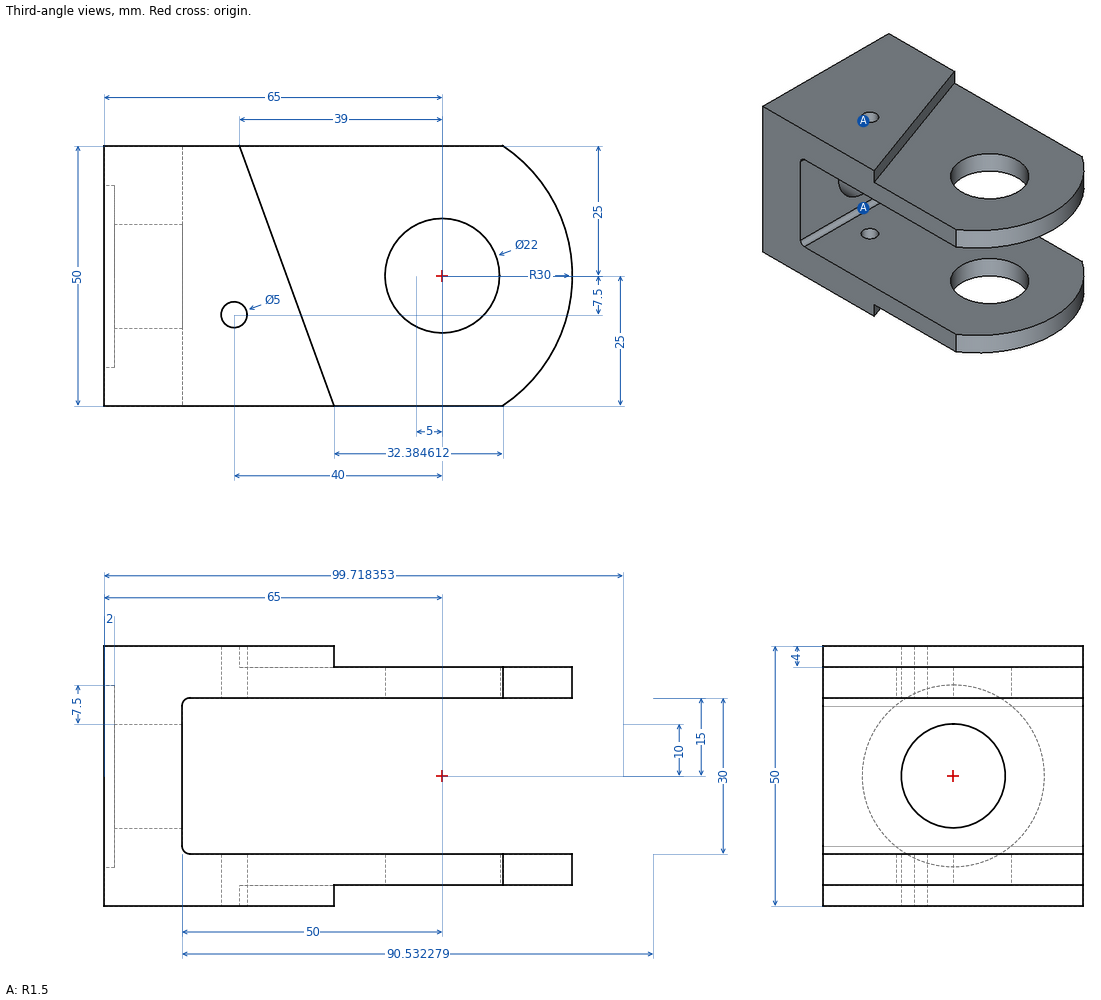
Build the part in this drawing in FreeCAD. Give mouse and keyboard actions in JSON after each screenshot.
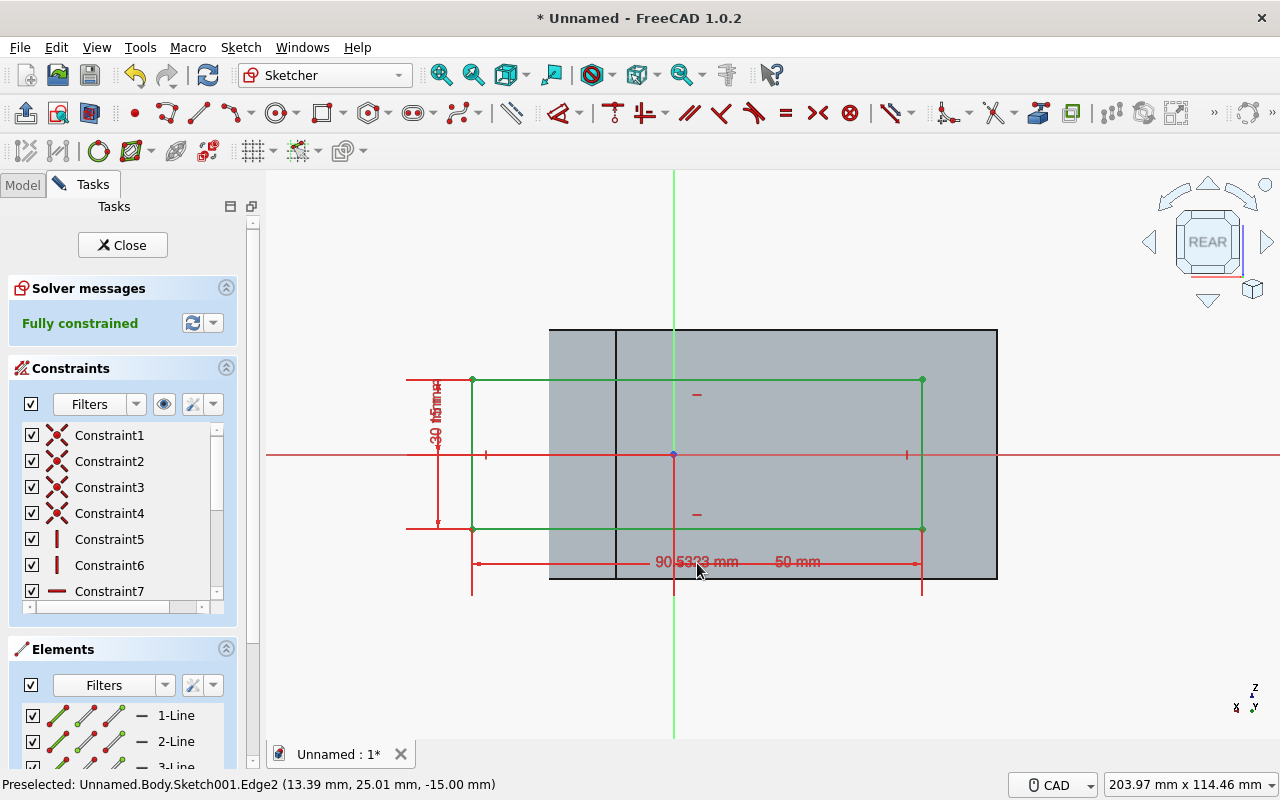
{"action": "left_click", "coordinate": [123, 245]}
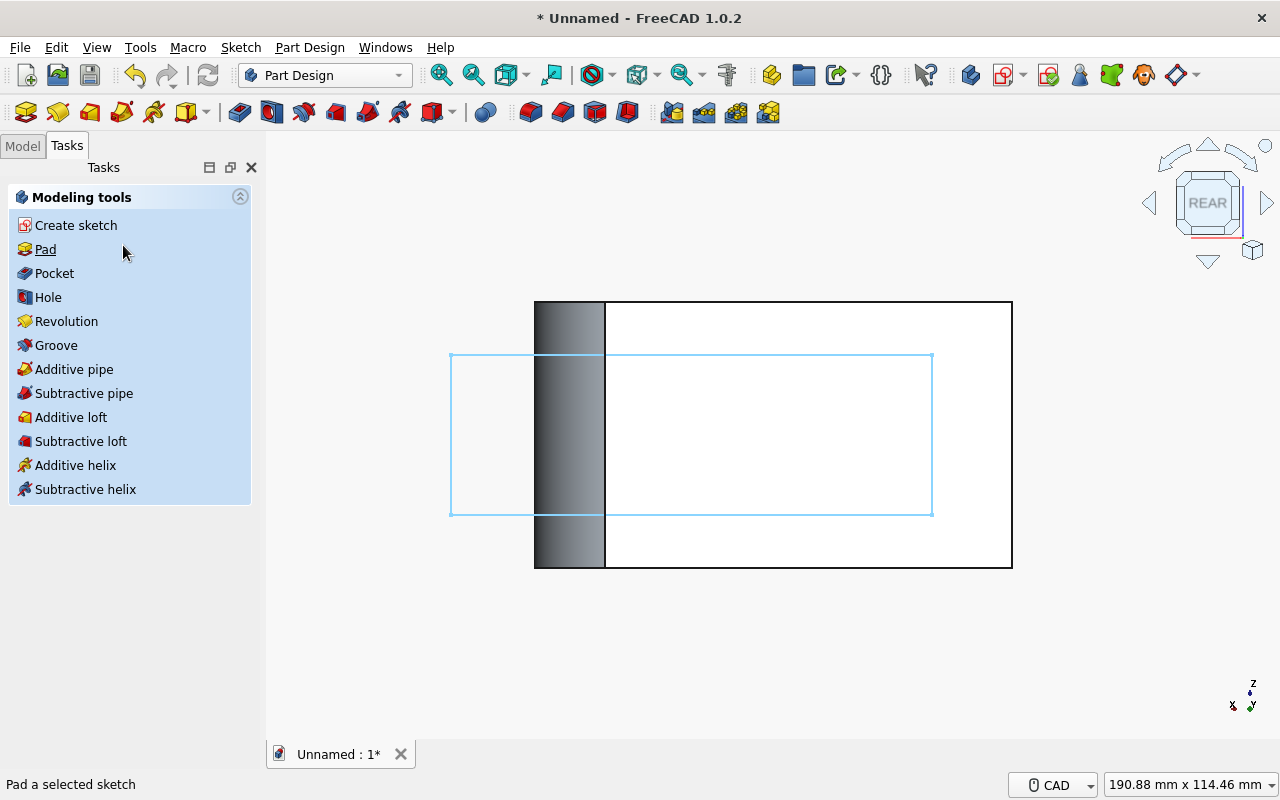
{"action": "left_click", "coordinate": [240, 112]}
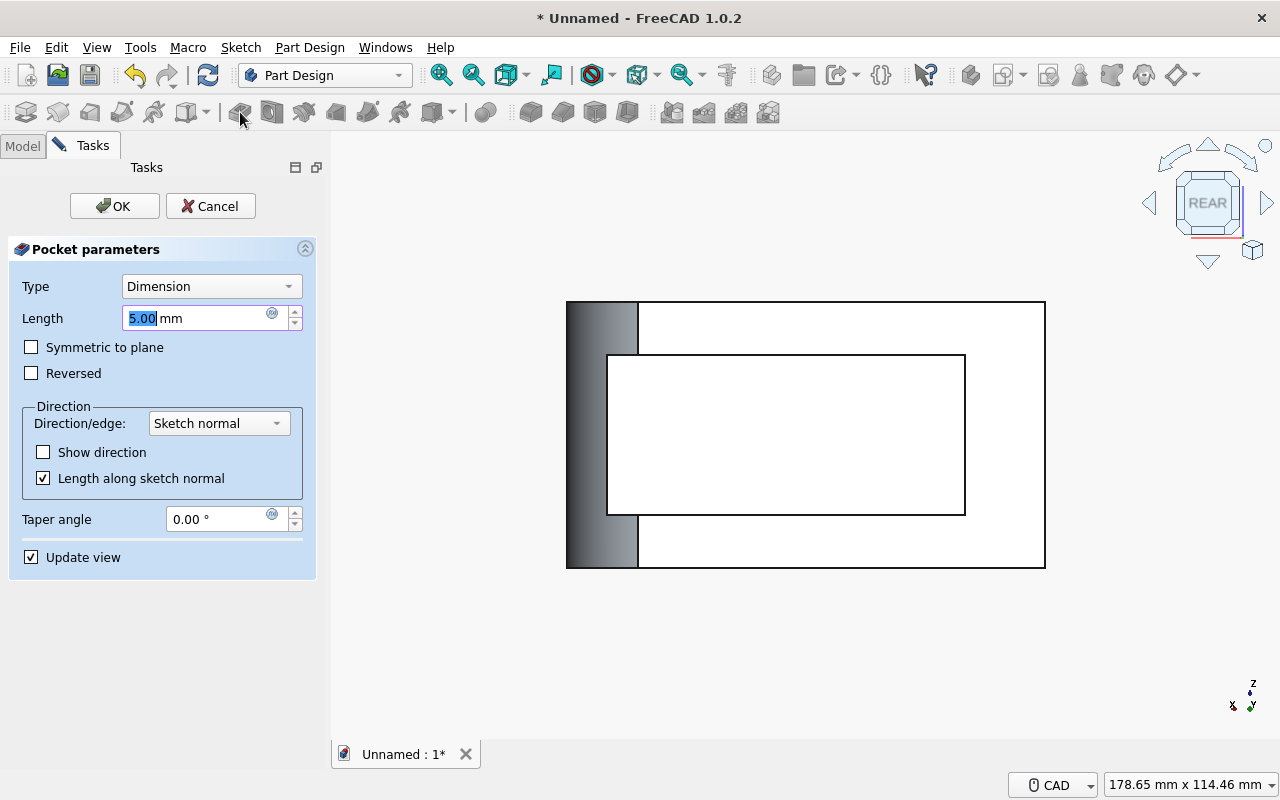
{"action": "left_click", "coordinate": [212, 286]}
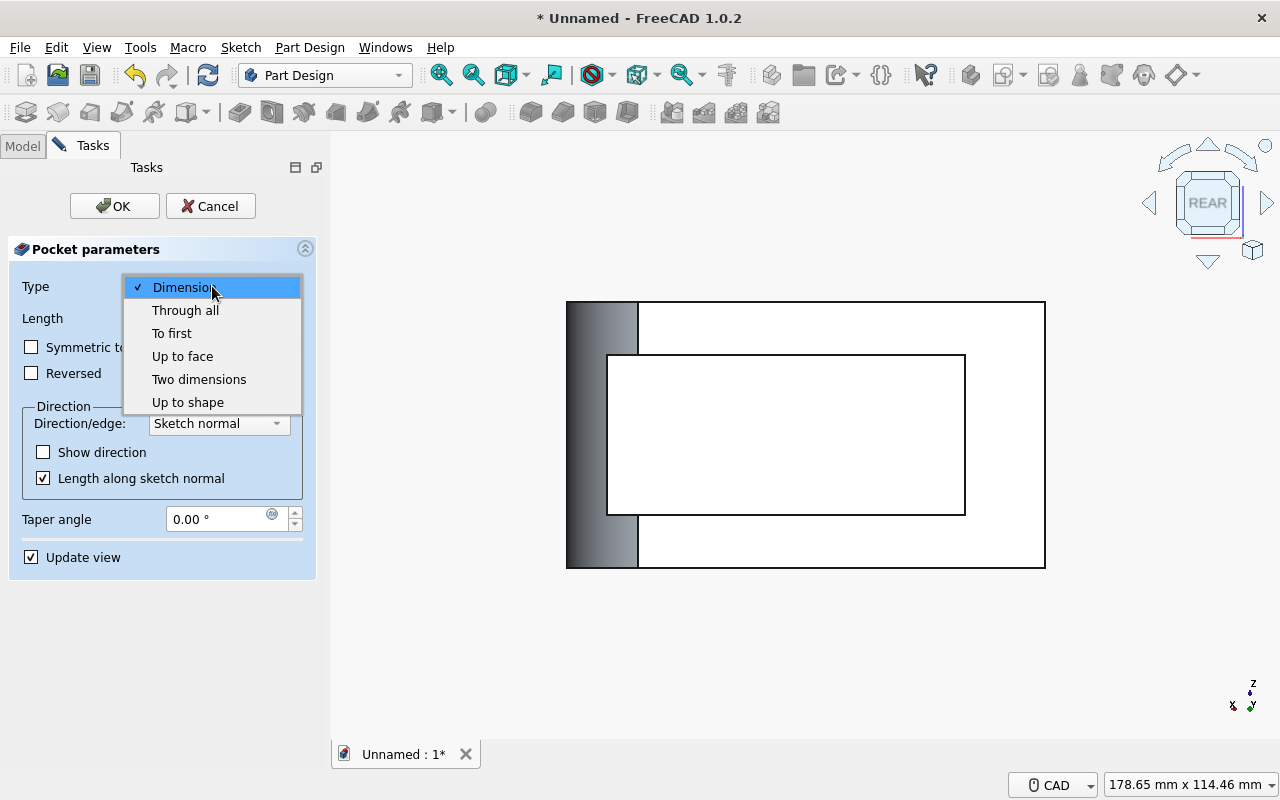
{"action": "left_click", "coordinate": [212, 310]}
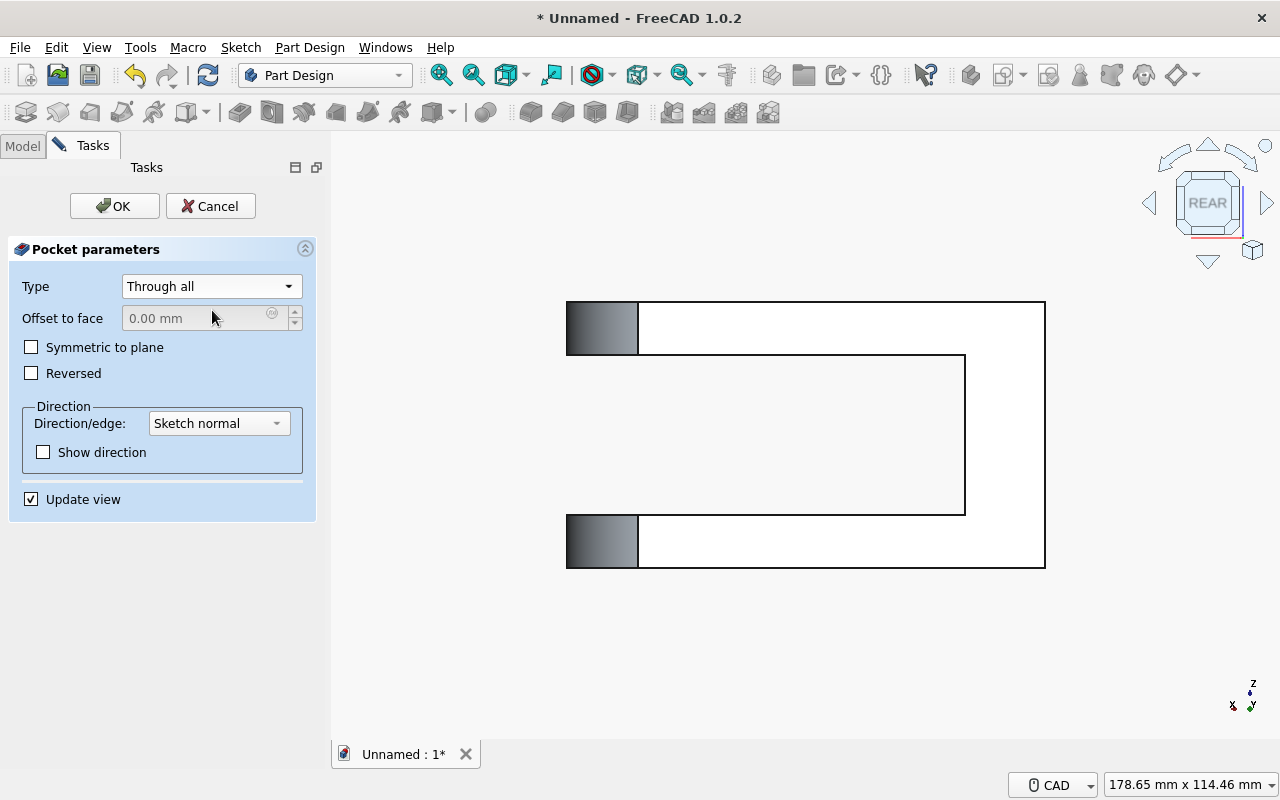
{"action": "left_click", "coordinate": [115, 206]}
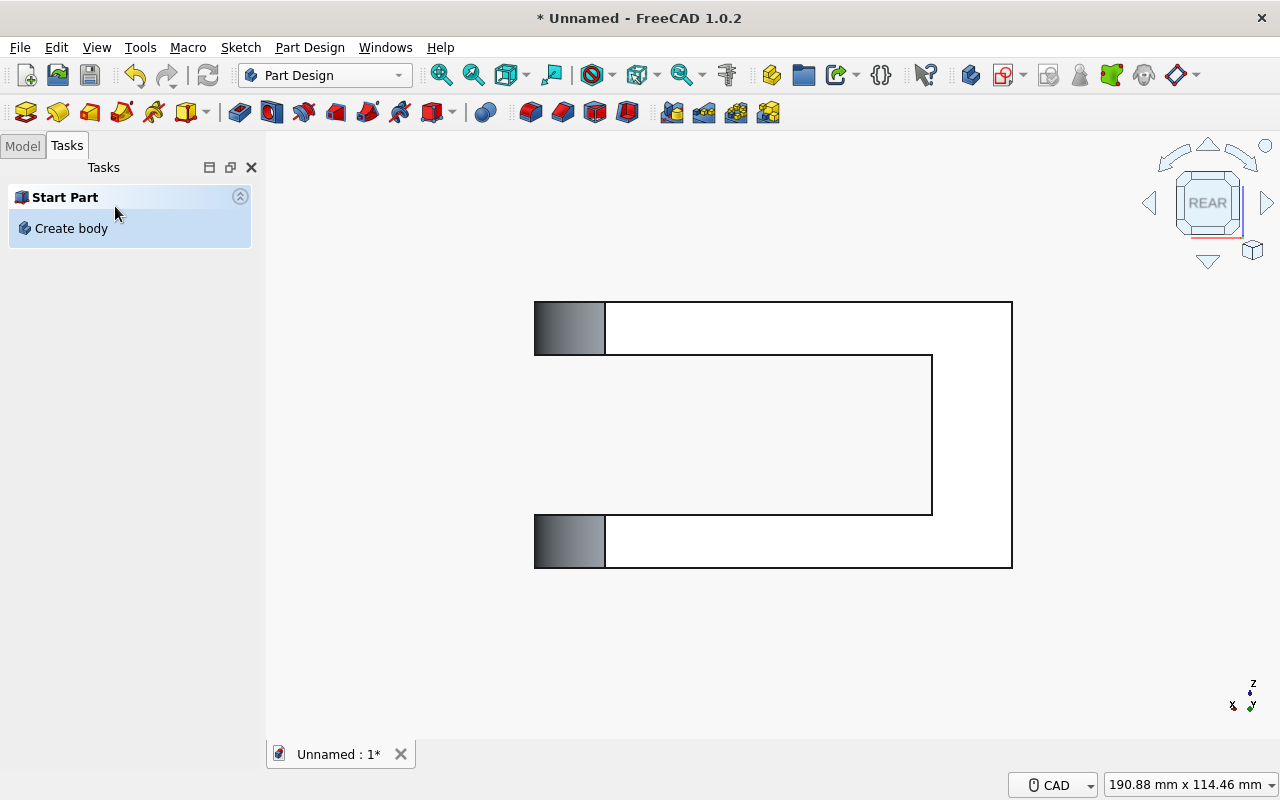
{"action": "key", "text": "0"}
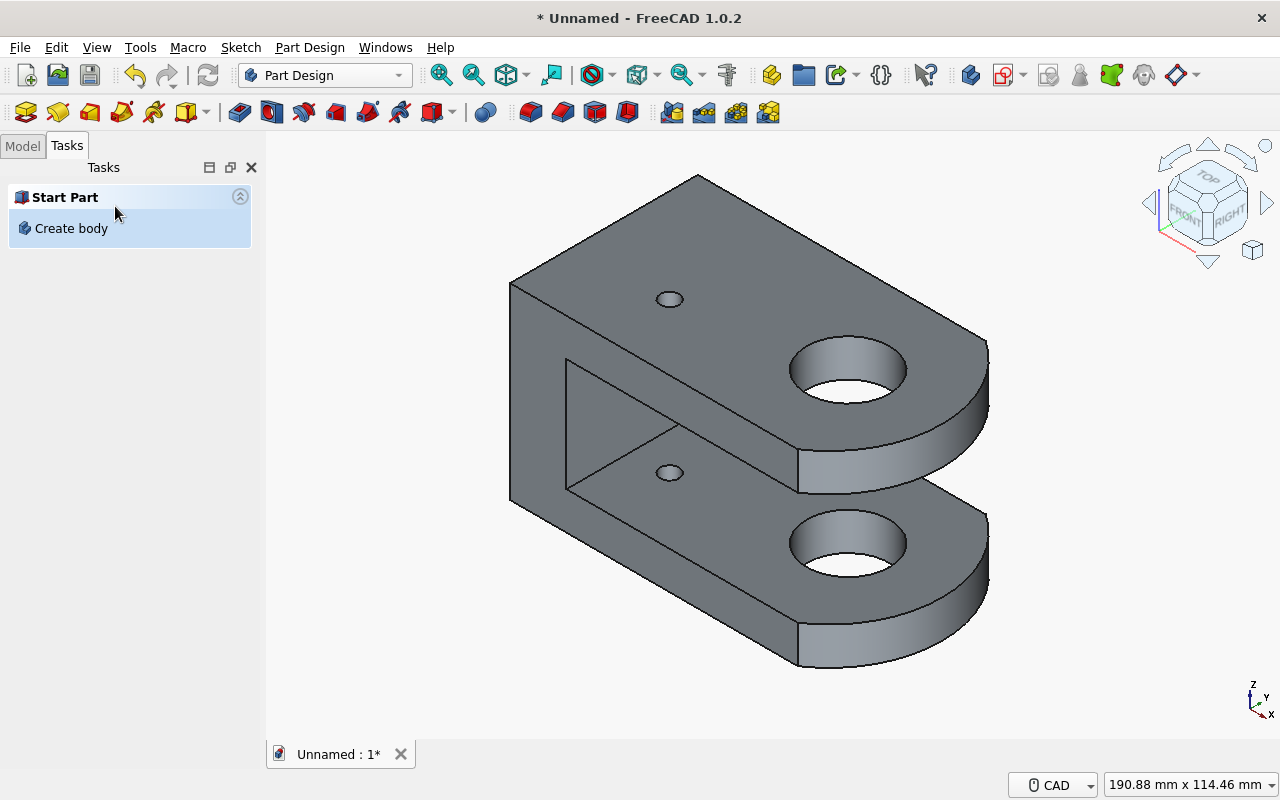
{"action": "left_click", "coordinate": [752, 282]}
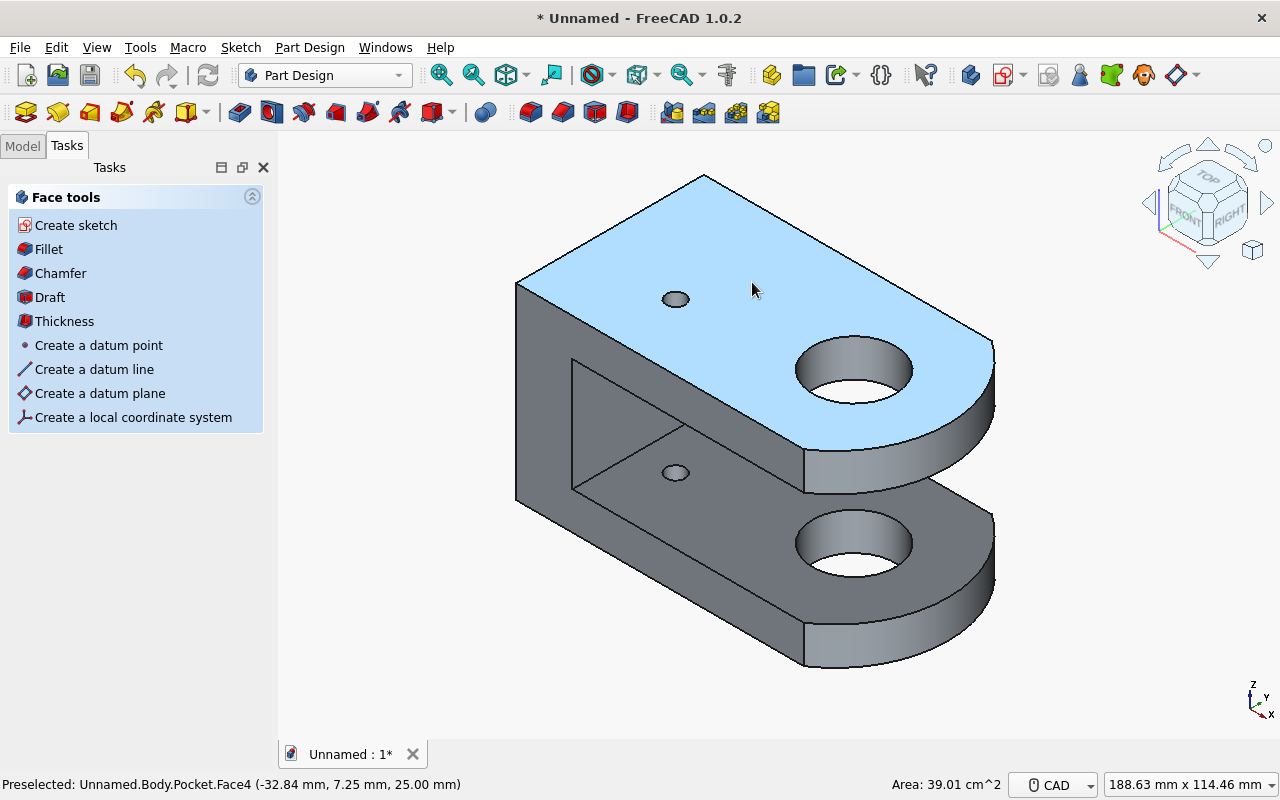
{"action": "left_click", "coordinate": [1004, 76]}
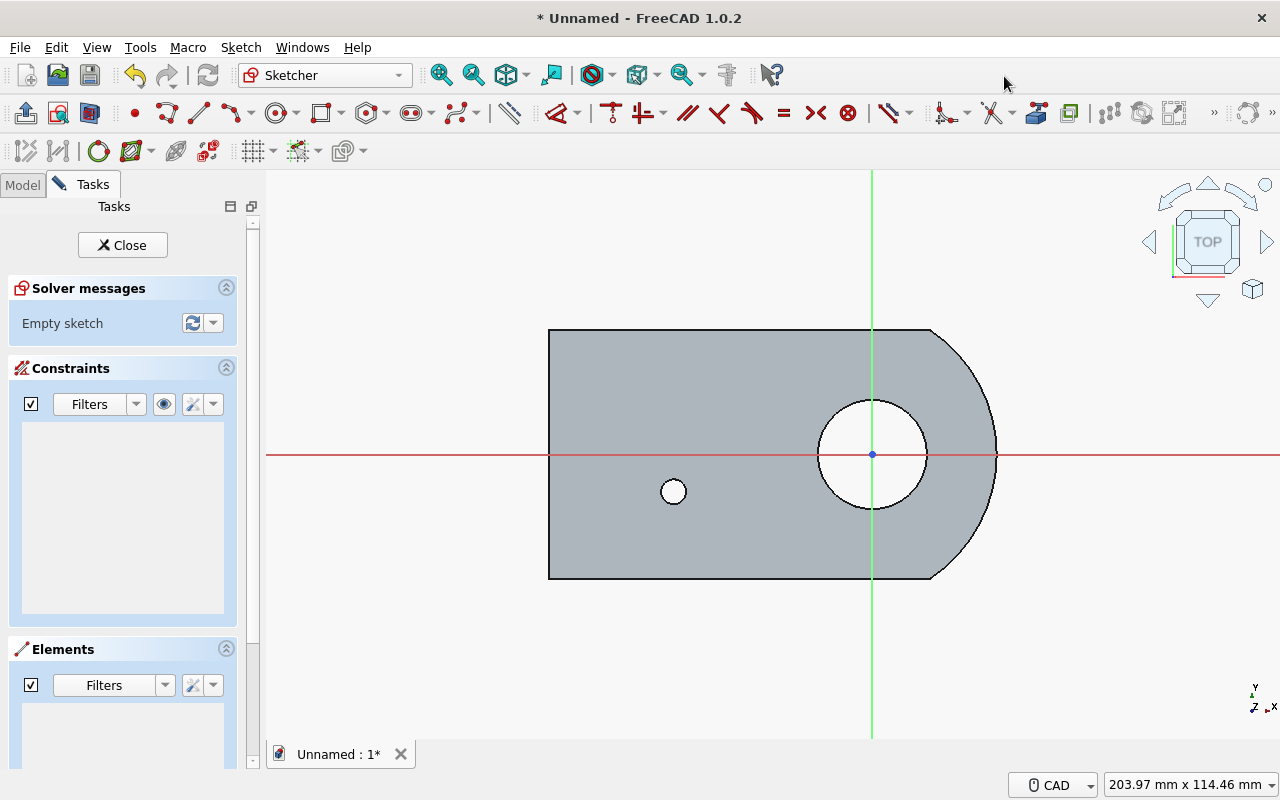
{"action": "scroll", "coordinate": [1108, 454], "scroll_direction": "up", "scroll_amount": 2}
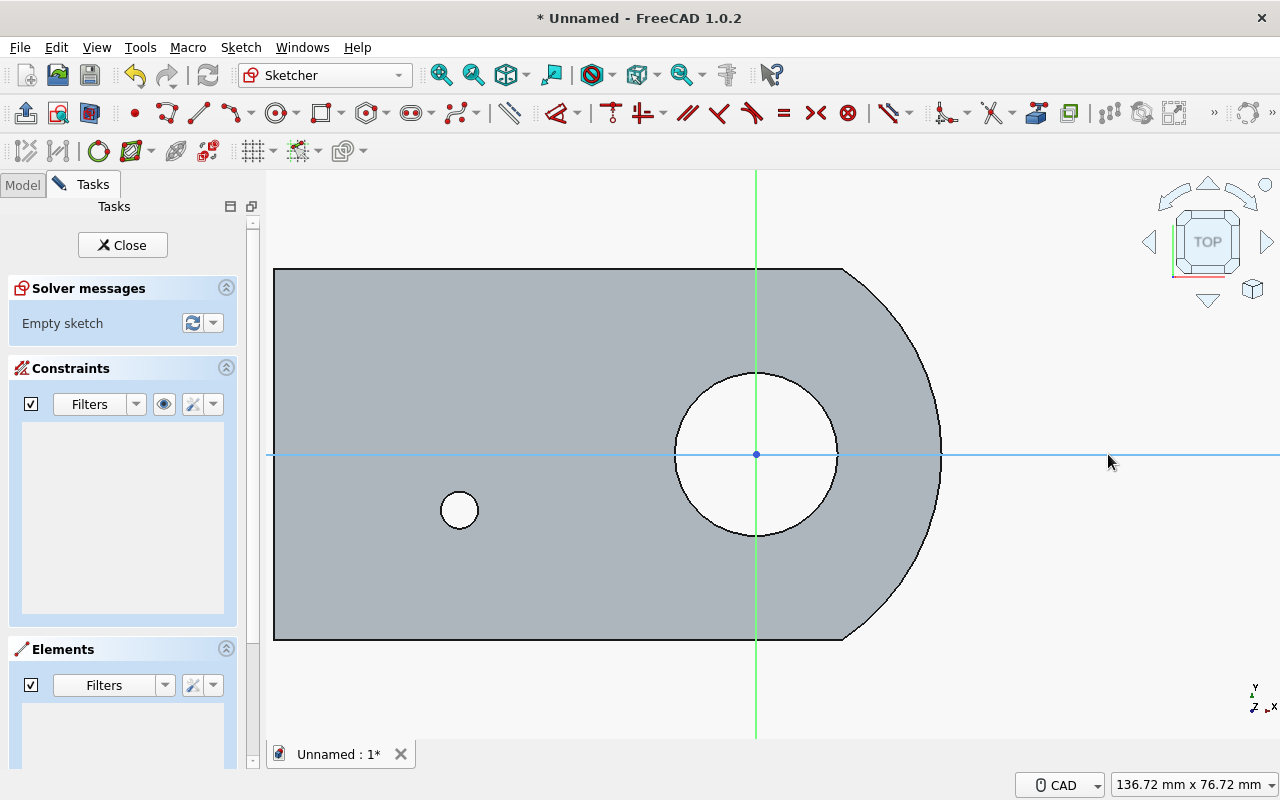
{"action": "left_click", "coordinate": [168, 114]}